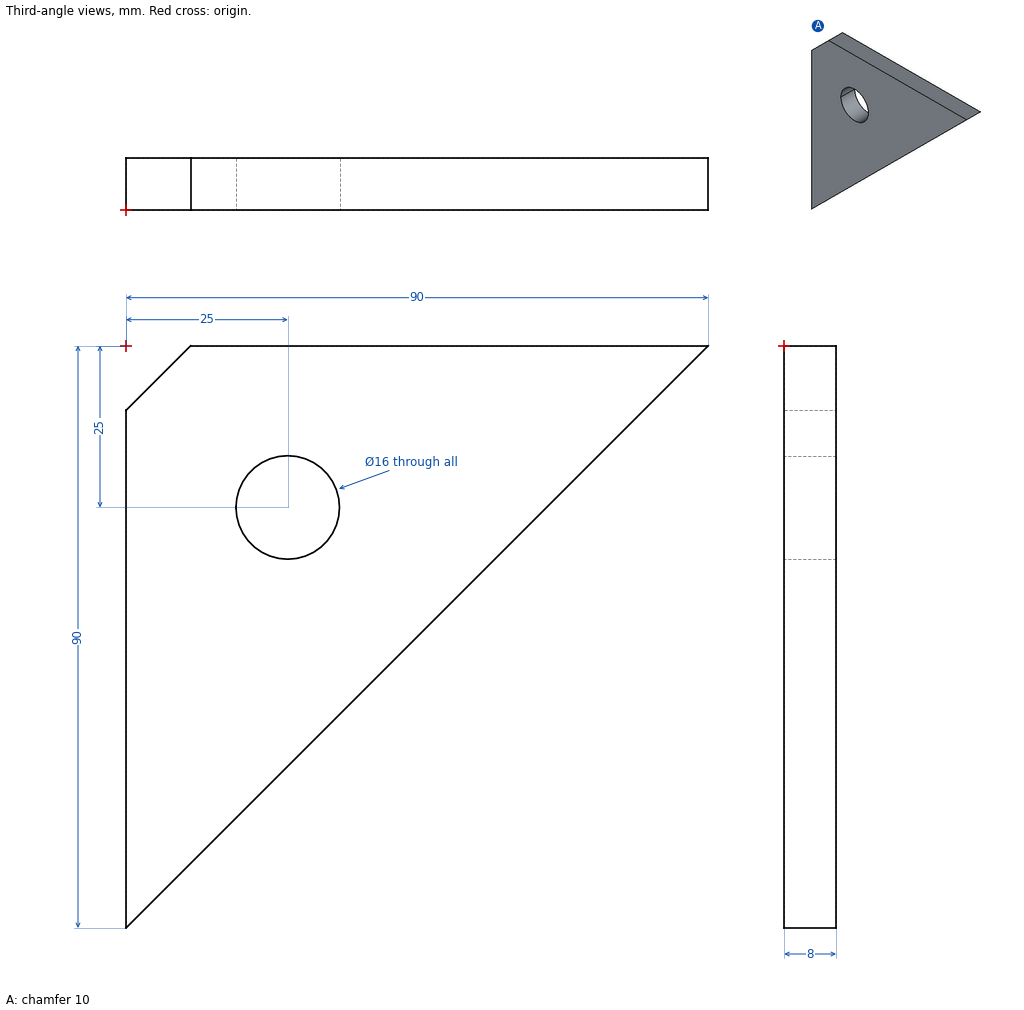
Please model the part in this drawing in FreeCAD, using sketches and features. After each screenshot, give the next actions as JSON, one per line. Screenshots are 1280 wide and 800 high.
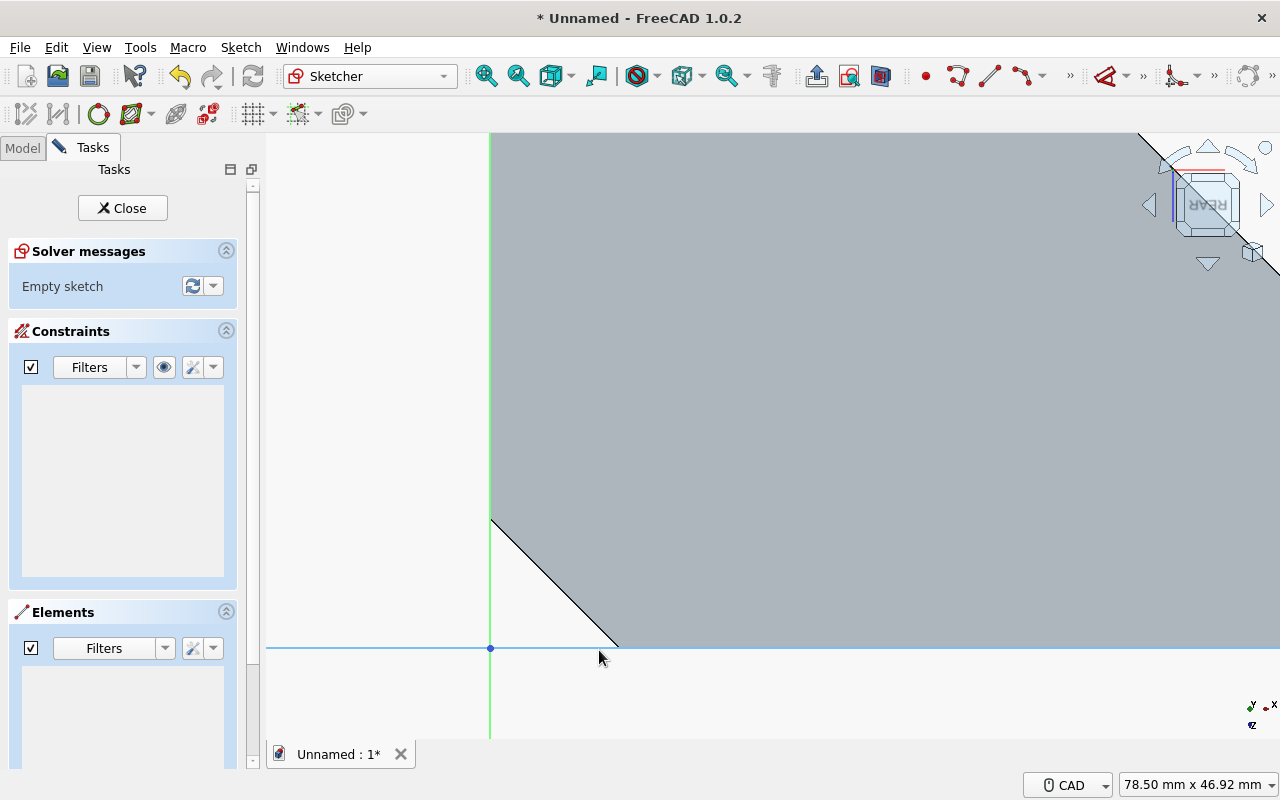
{"action": "key", "text": "g c"}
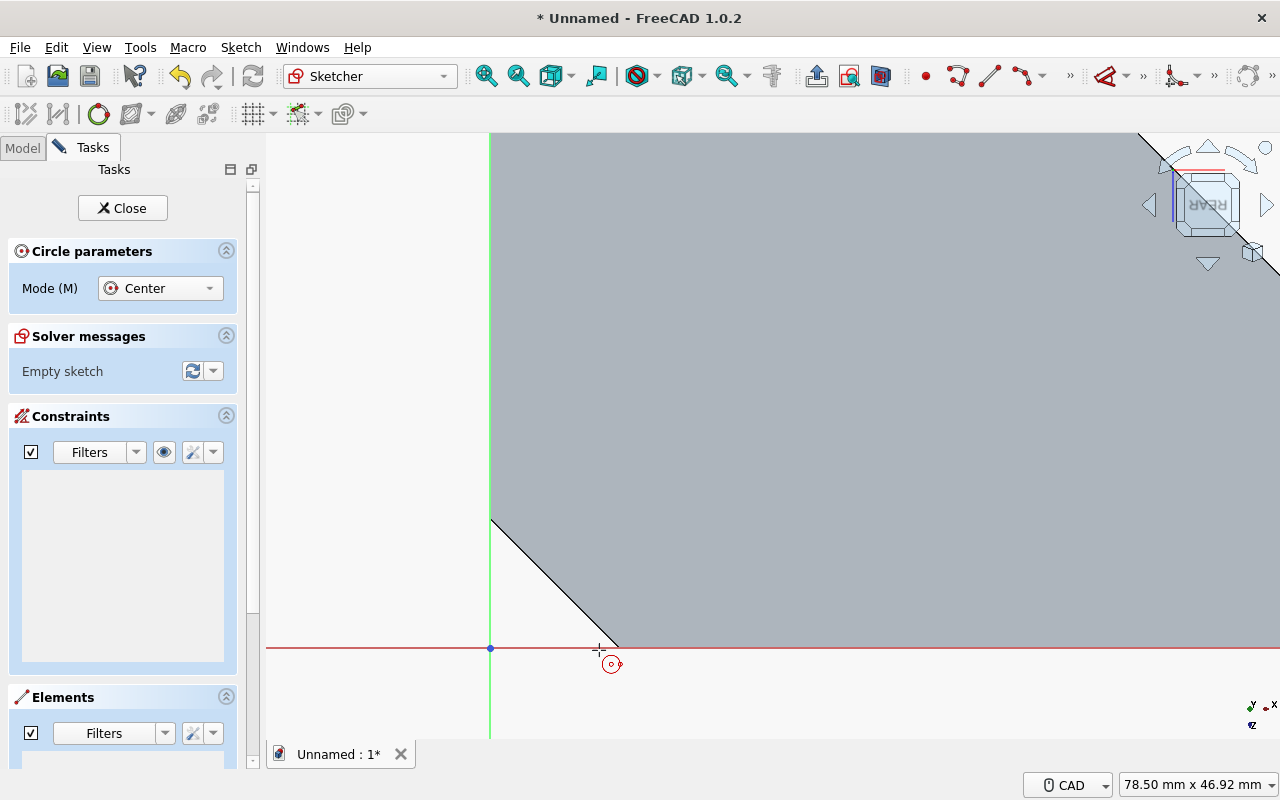
{"action": "left_click", "coordinate": [813, 325]}
{"action": "mouse_move", "coordinate": [886, 252]}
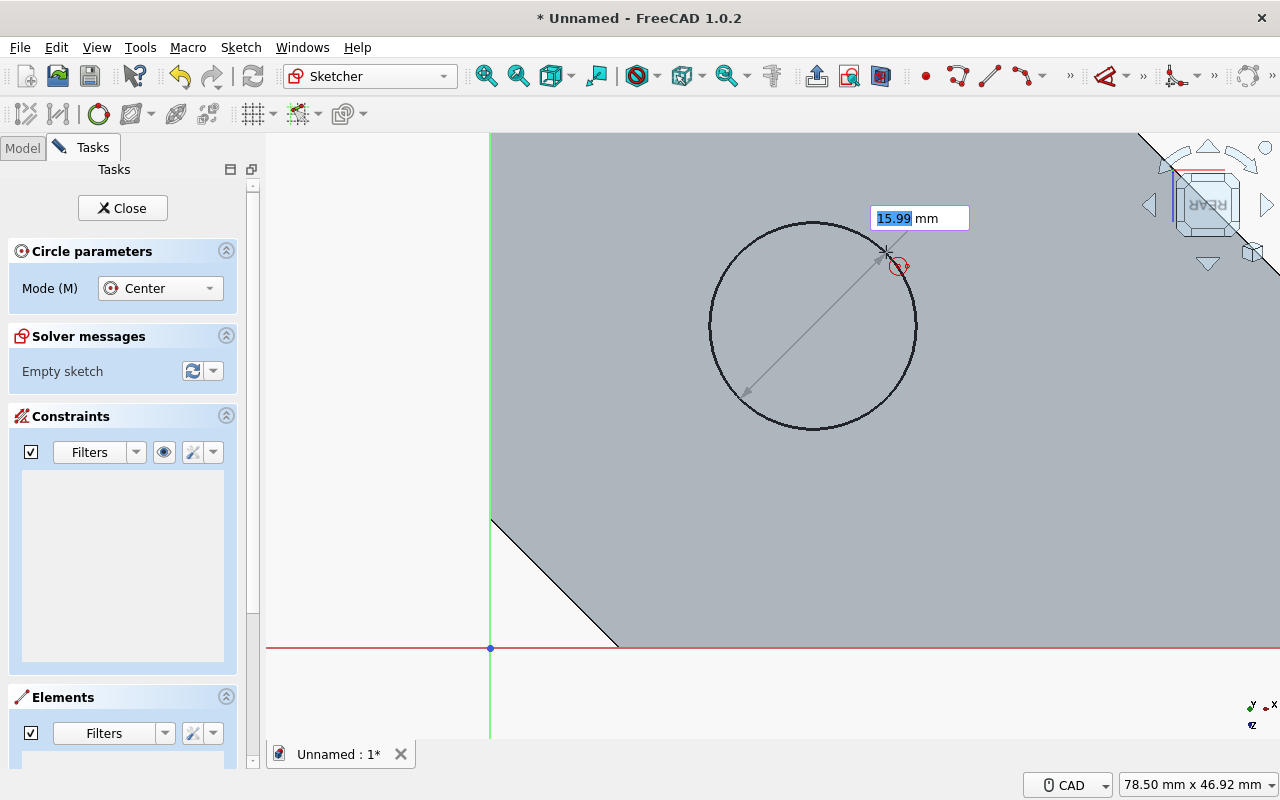
{"action": "type", "text": "16"}
{"action": "key", "text": "Return"}
{"action": "key", "text": "Escape"}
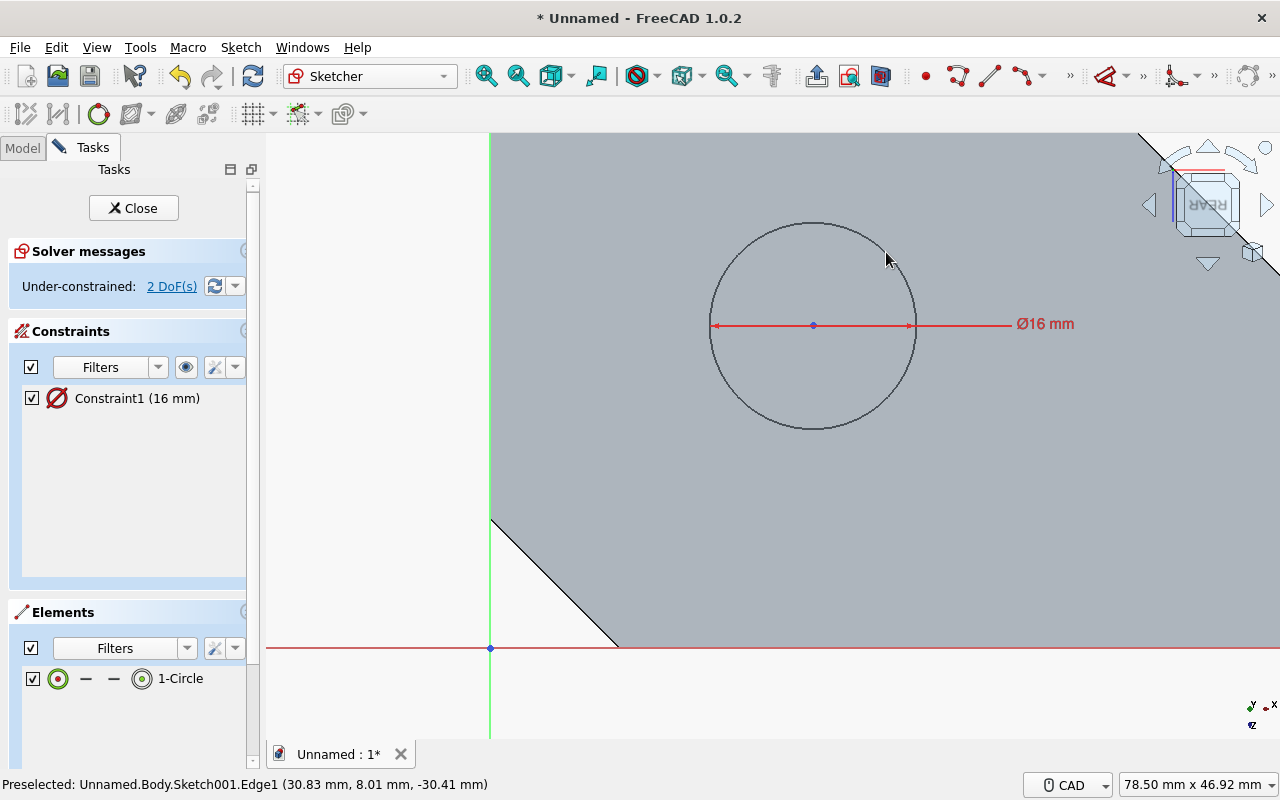
{"action": "key", "text": "d"}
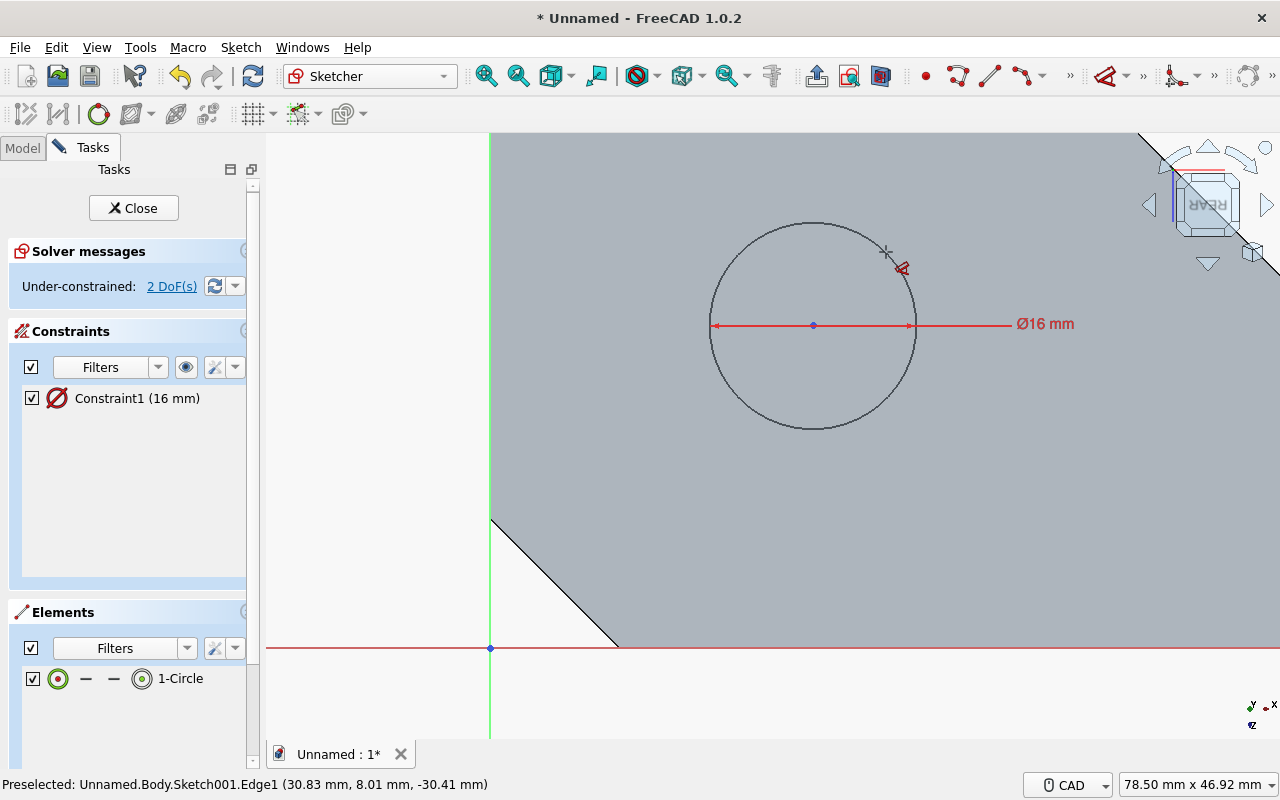
{"action": "left_click", "coordinate": [813, 326]}
{"action": "left_click", "coordinate": [652, 682]}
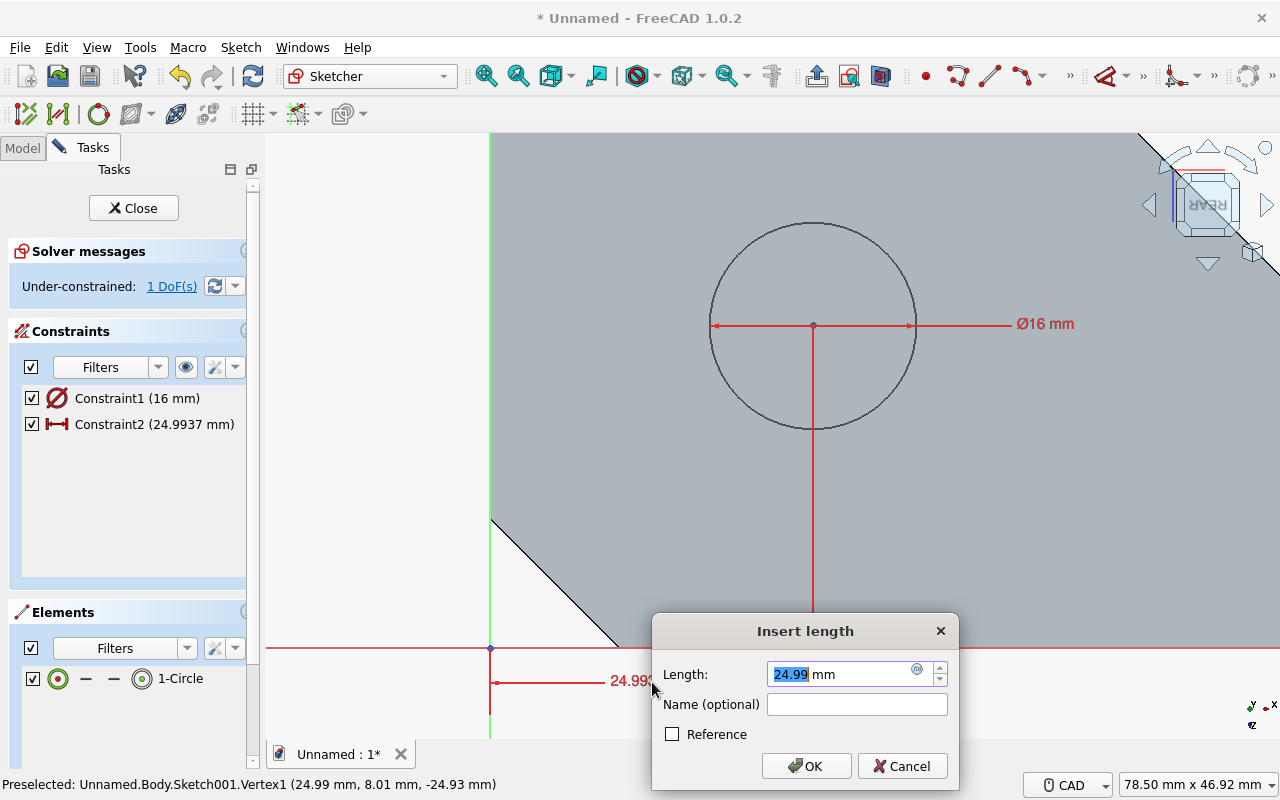
{"action": "type", "text": "25"}
{"action": "key", "text": "Return"}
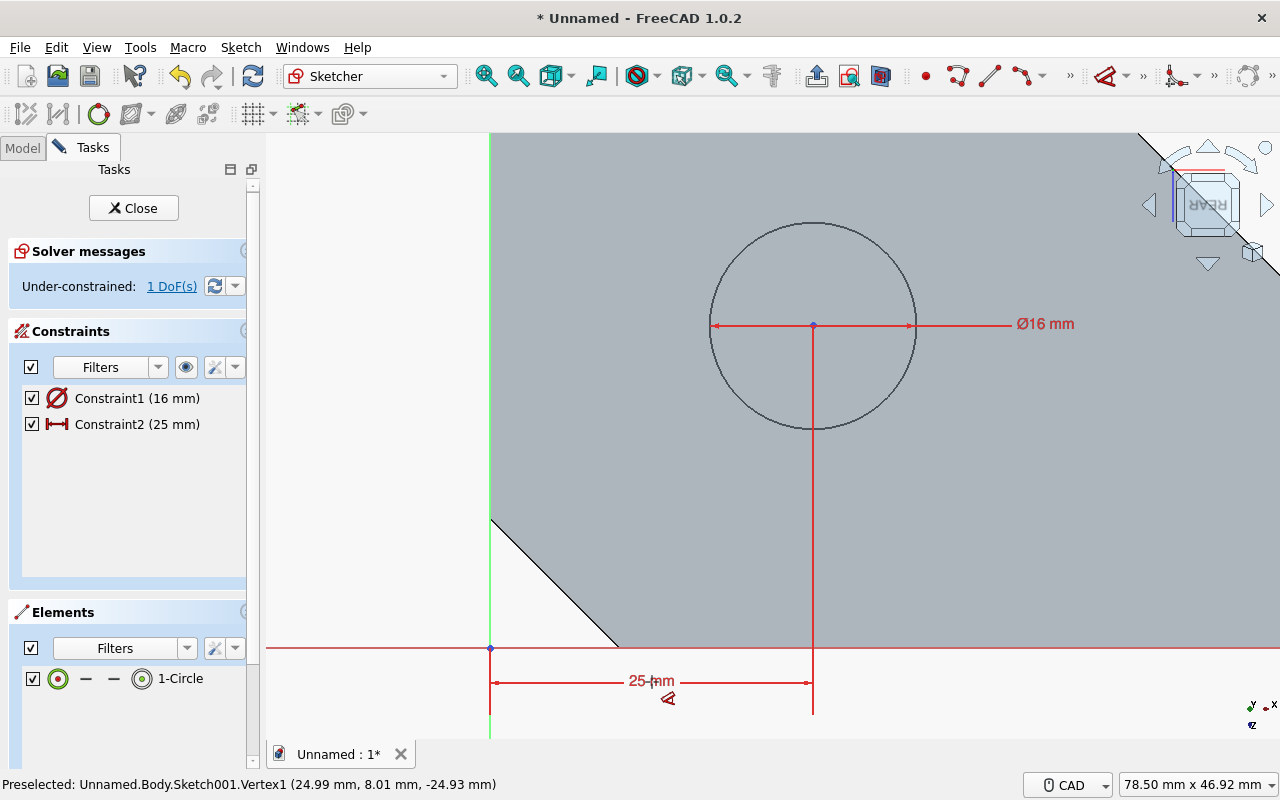
{"action": "left_click", "coordinate": [813, 326]}
{"action": "left_click", "coordinate": [456, 487]}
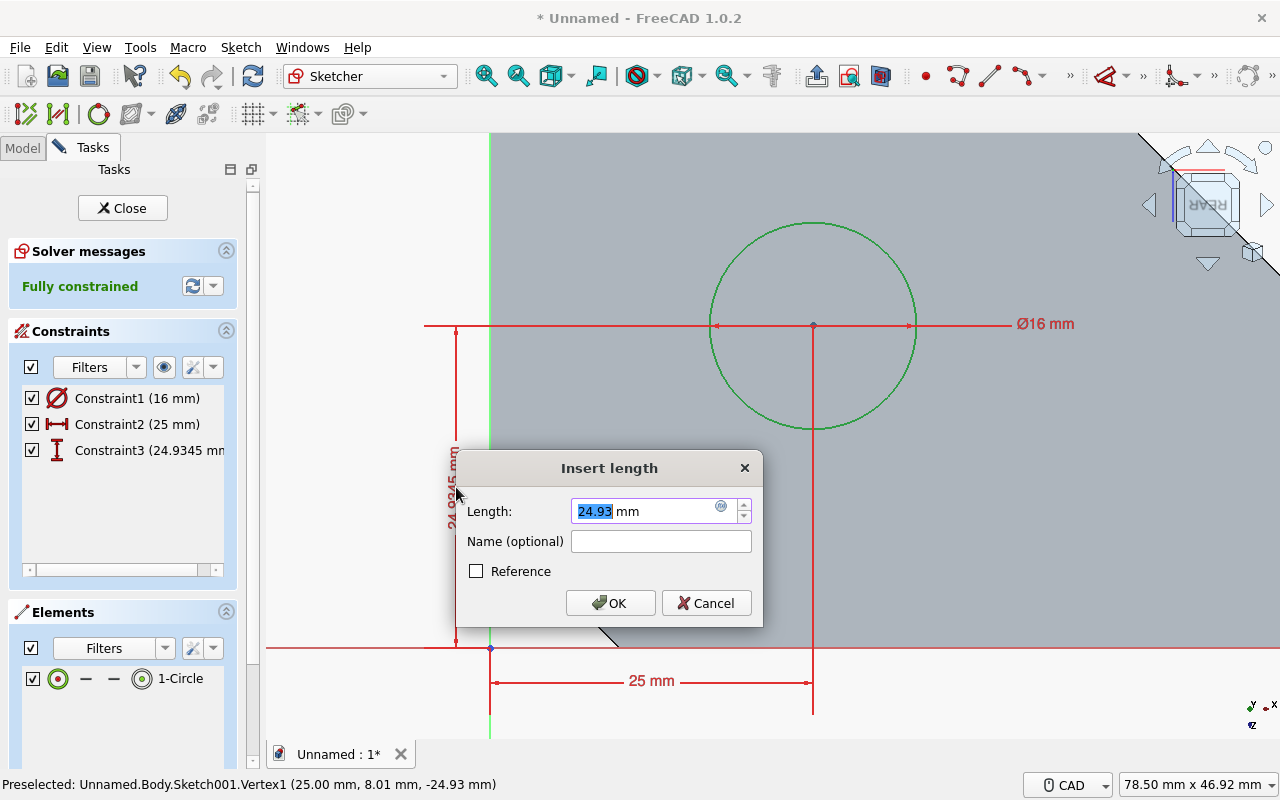
{"action": "type", "text": "25"}
{"action": "key", "text": "Return"}
{"action": "key", "text": "Escape"}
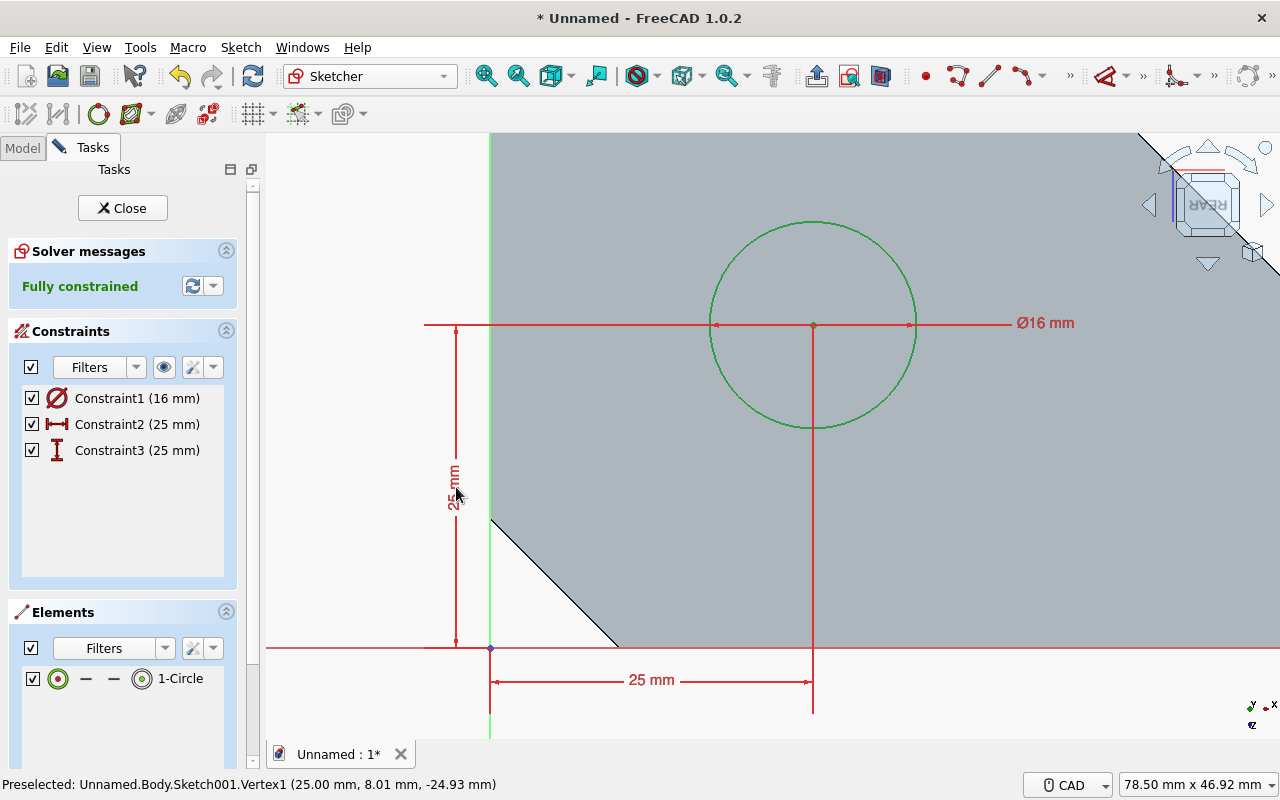
{"action": "left_click", "coordinate": [123, 208]}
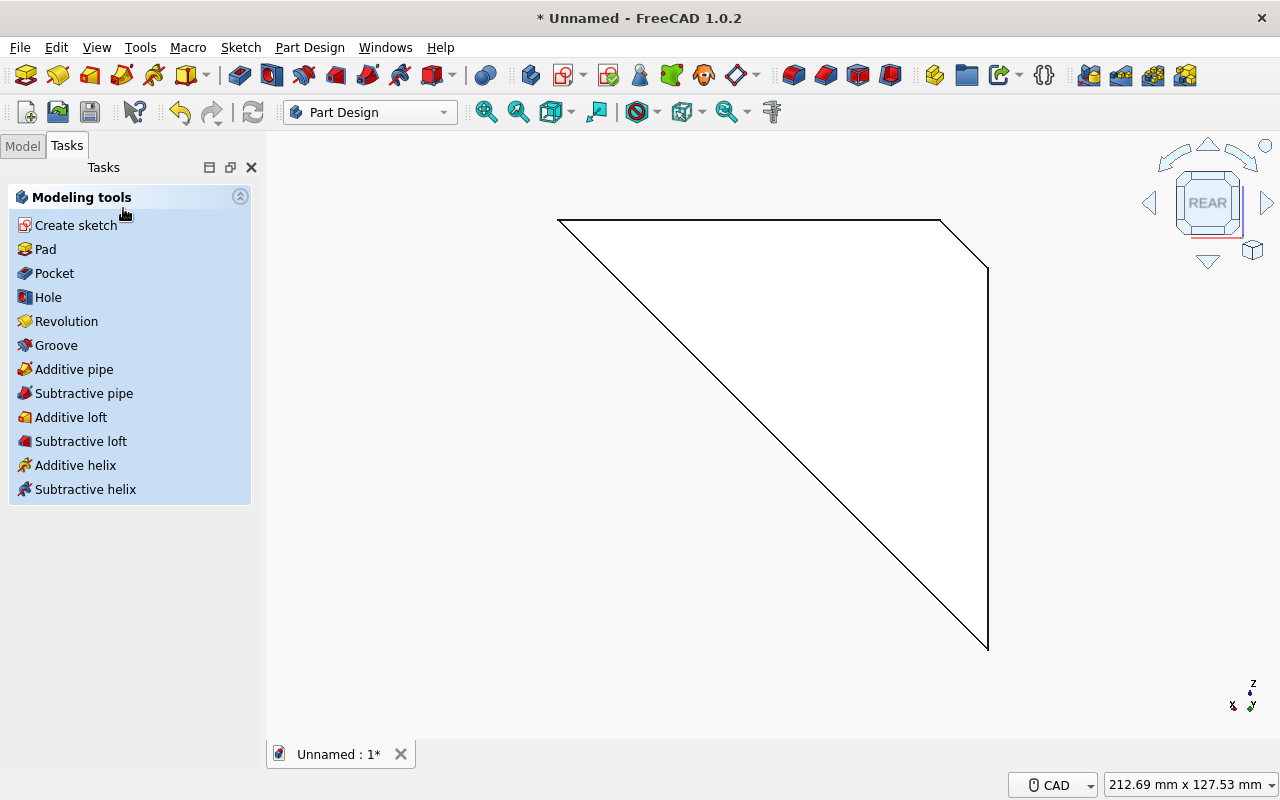
{"action": "left_click", "coordinate": [272, 76]}